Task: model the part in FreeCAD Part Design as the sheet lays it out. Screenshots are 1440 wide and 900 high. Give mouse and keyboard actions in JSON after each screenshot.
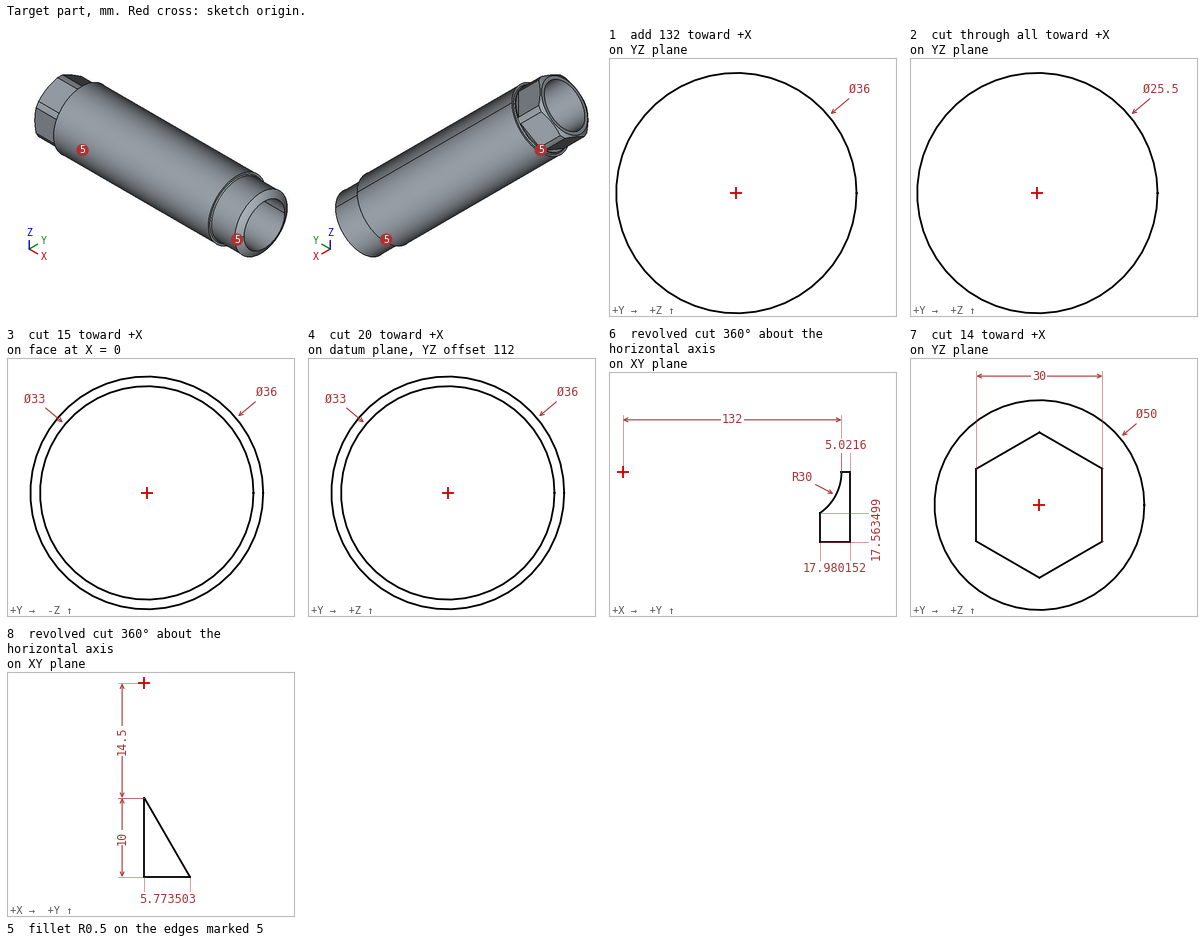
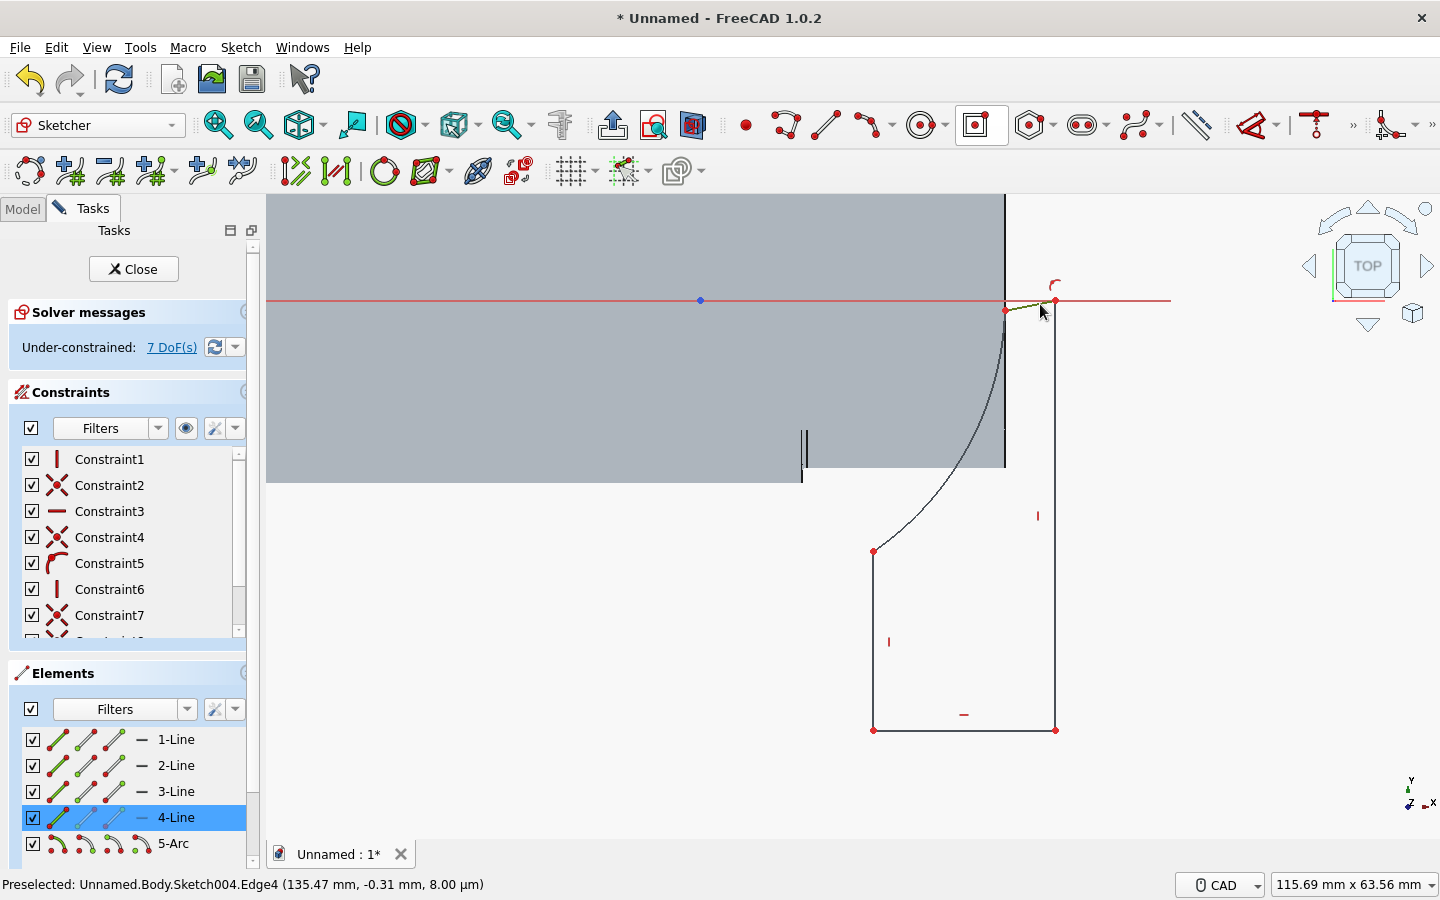
{"action": "key", "text": "h"}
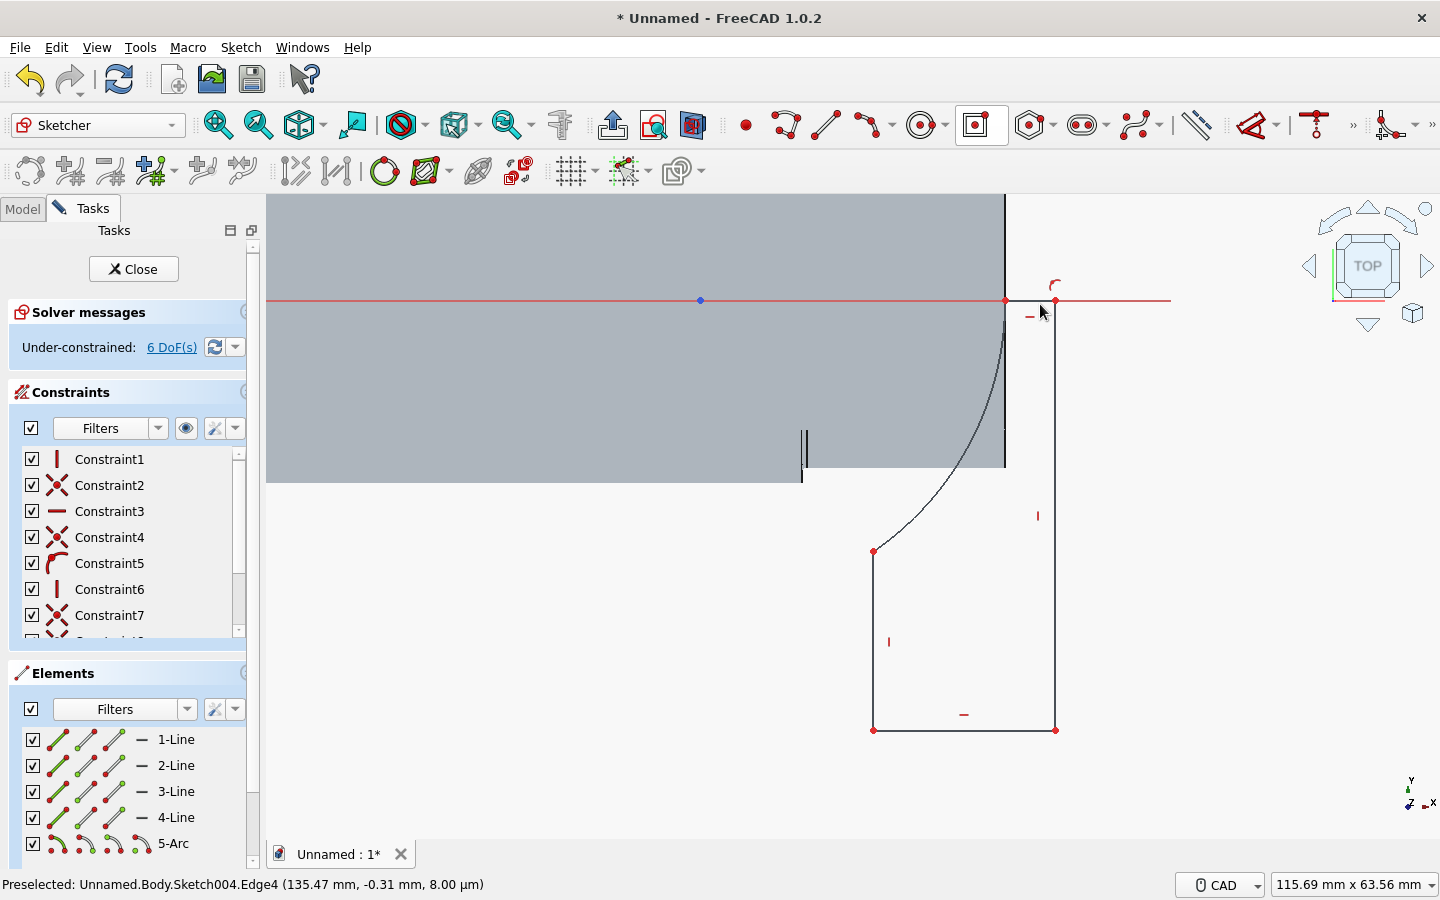
{"action": "left_click", "coordinate": [701, 301]}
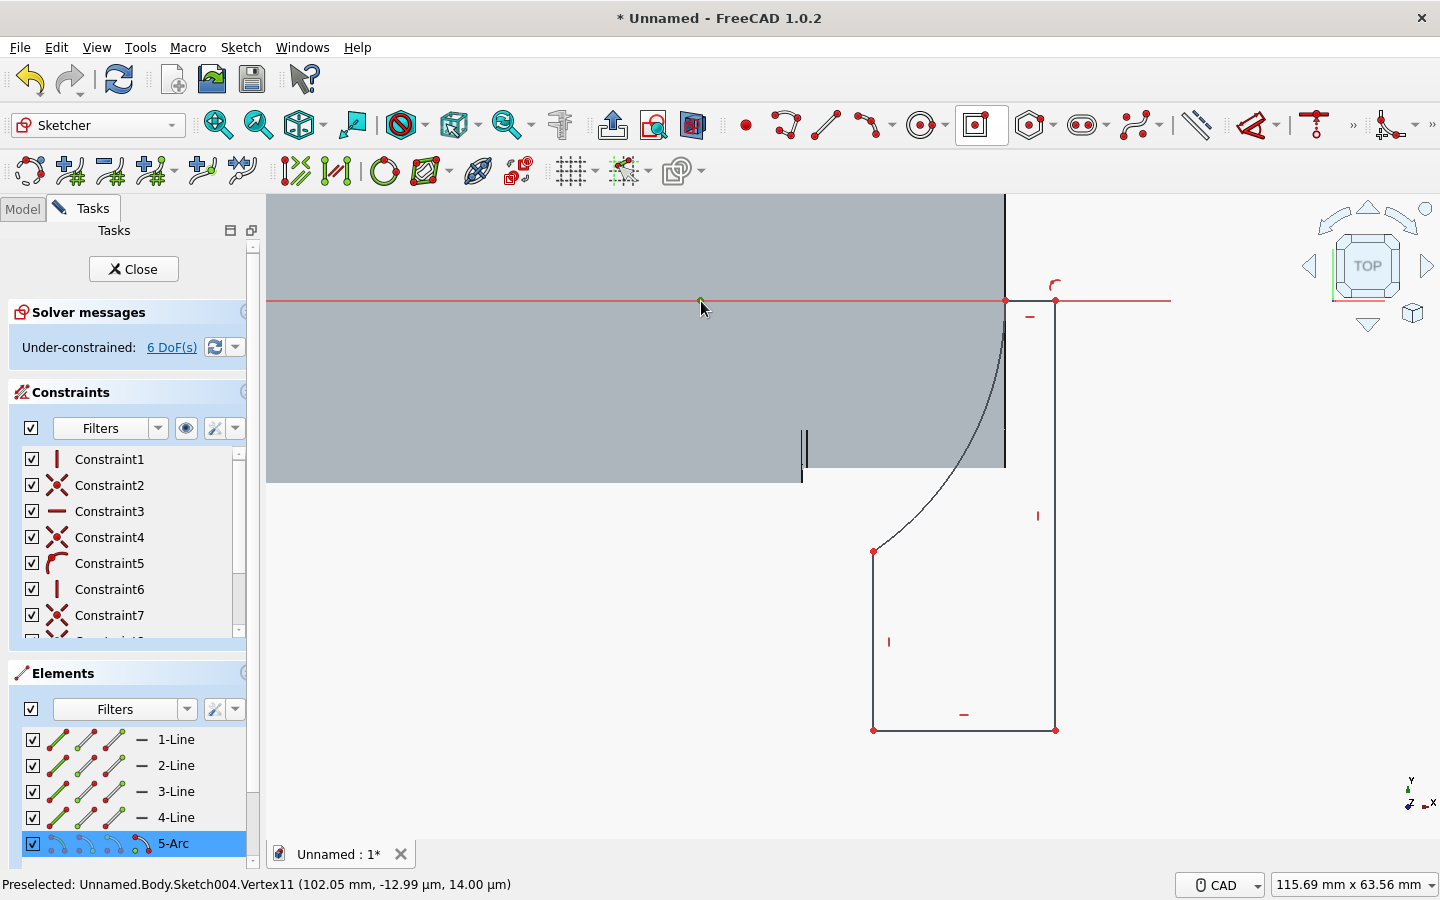
{"action": "left_click", "coordinate": [364, 301]}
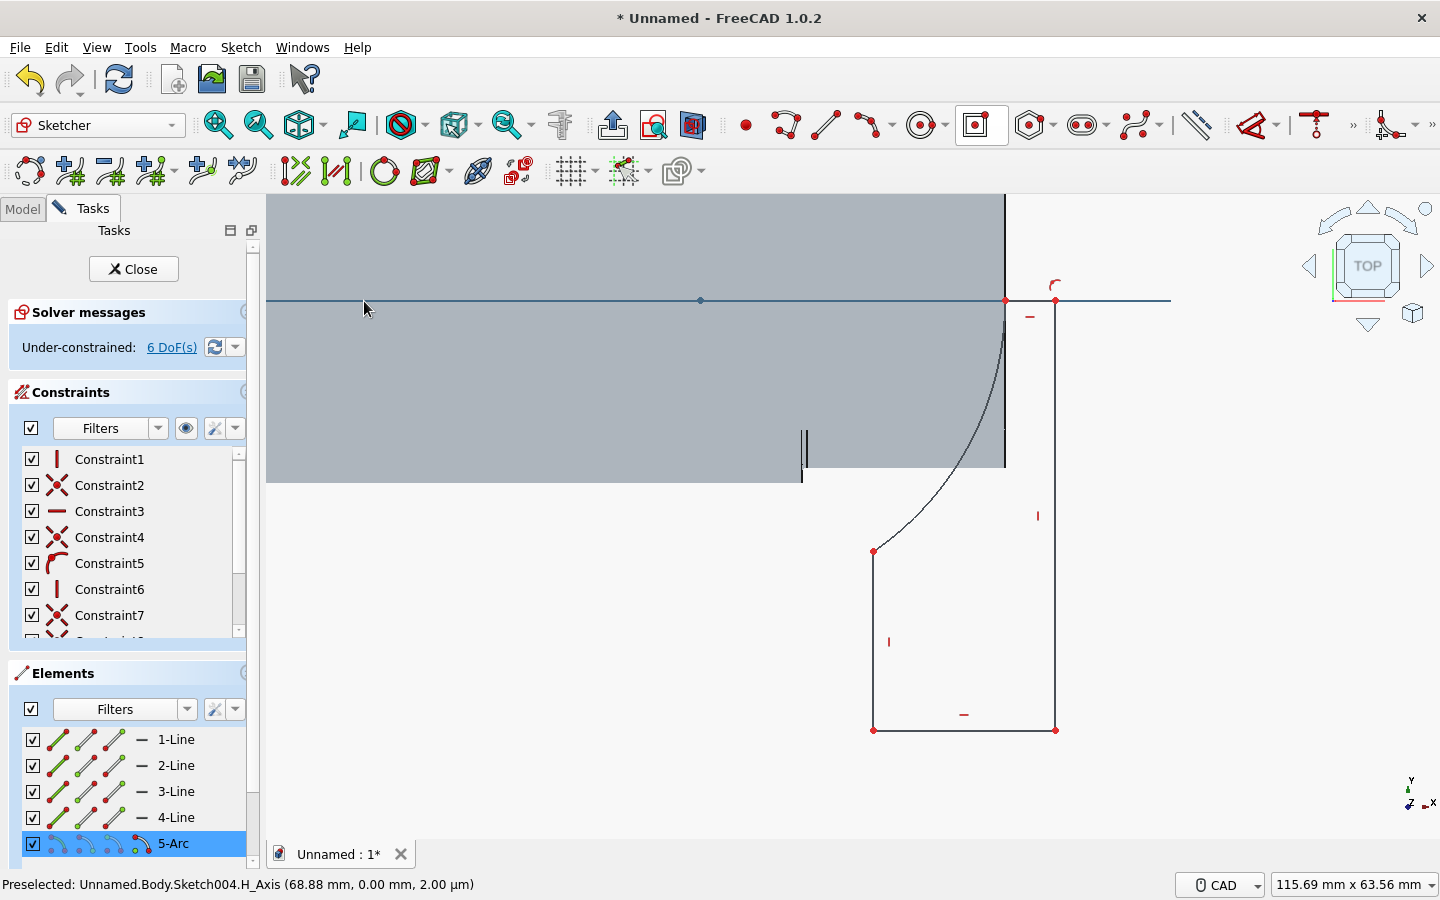
{"action": "left_click", "coordinate": [1314, 126]}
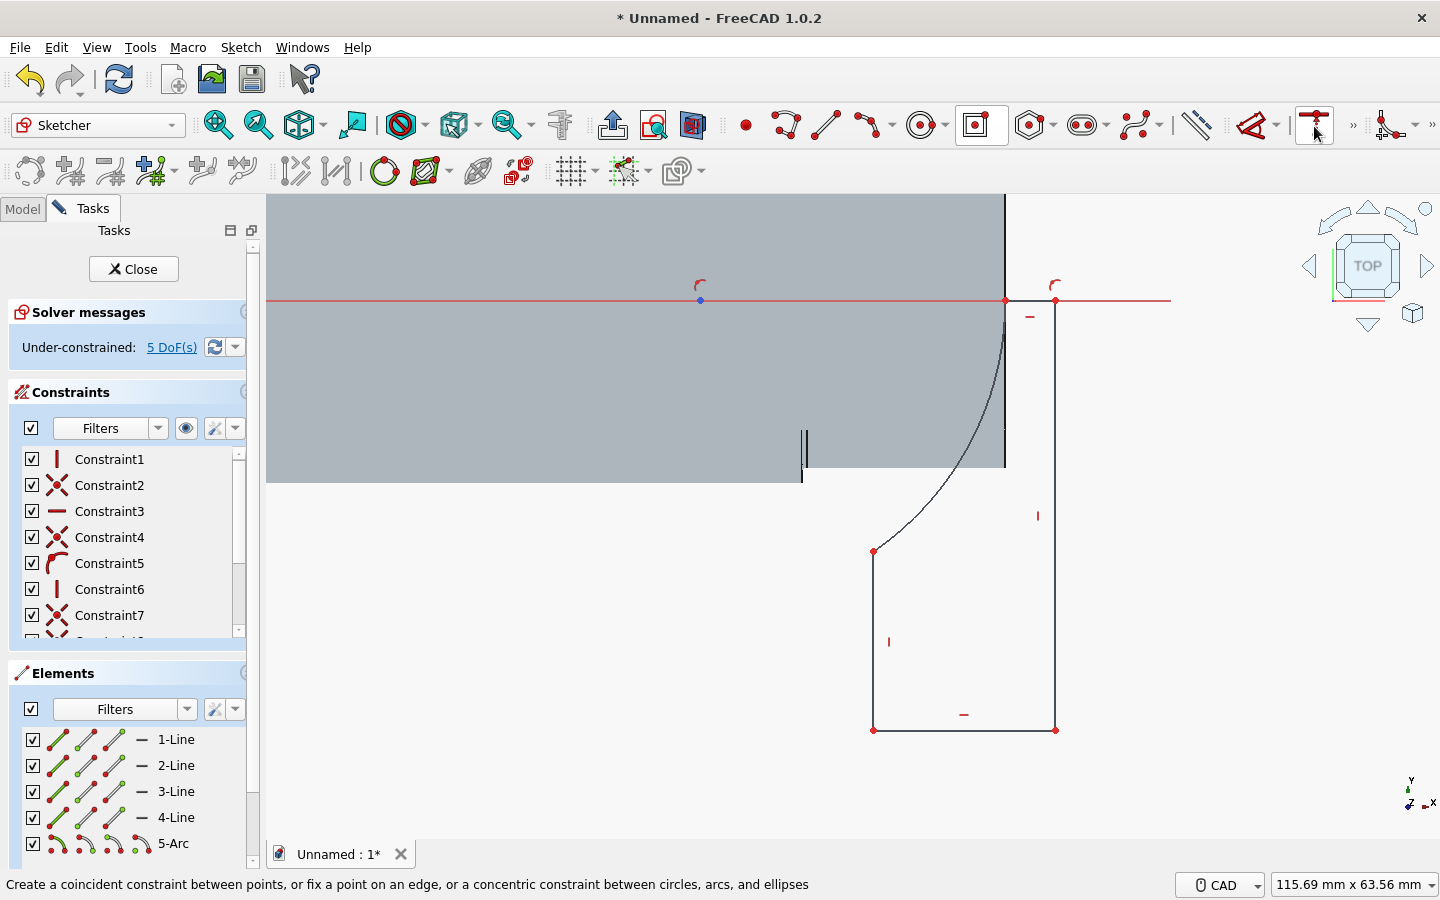
{"action": "left_click", "coordinate": [938, 492]}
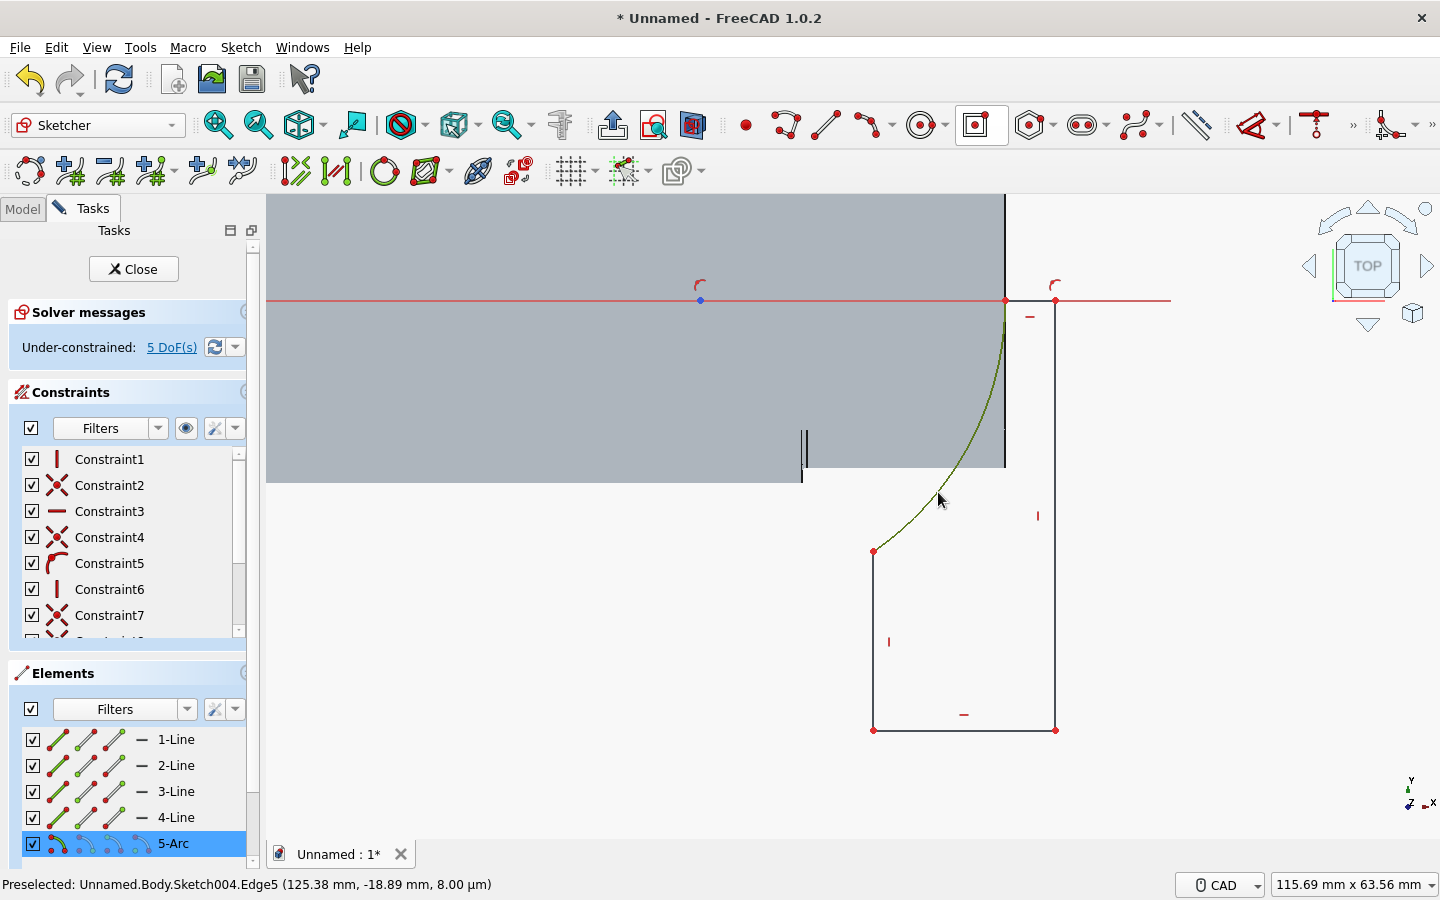
{"action": "key", "text": "k r"}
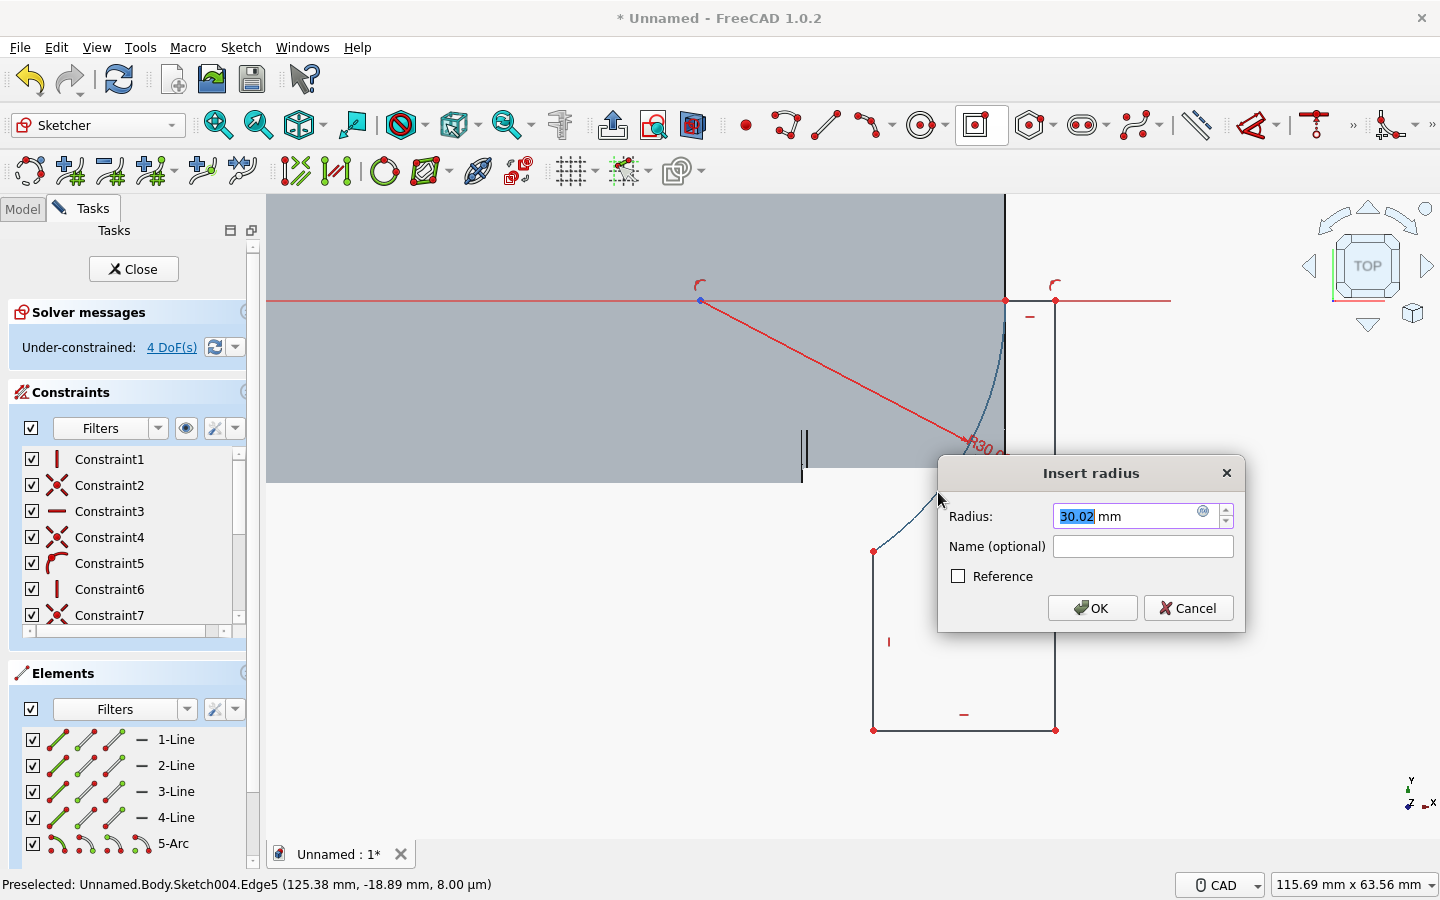
{"action": "type", "text": "30"}
{"action": "key", "text": "Return"}